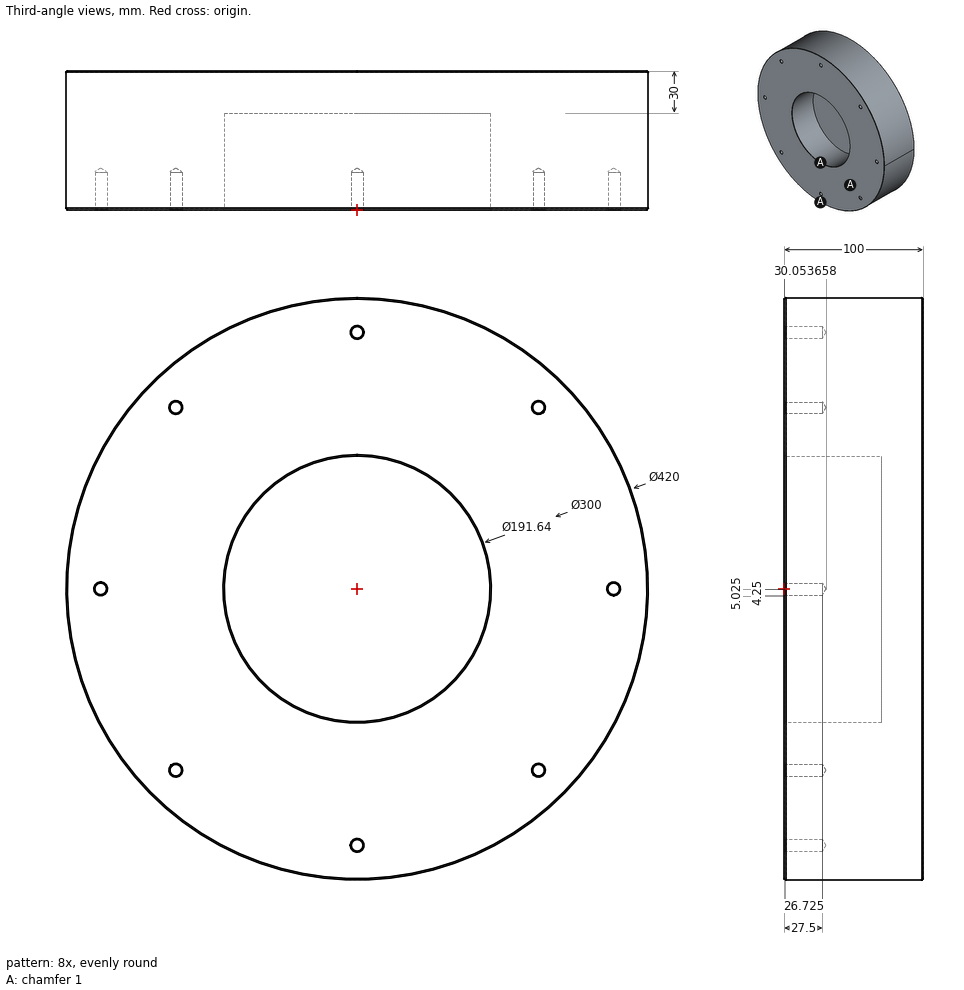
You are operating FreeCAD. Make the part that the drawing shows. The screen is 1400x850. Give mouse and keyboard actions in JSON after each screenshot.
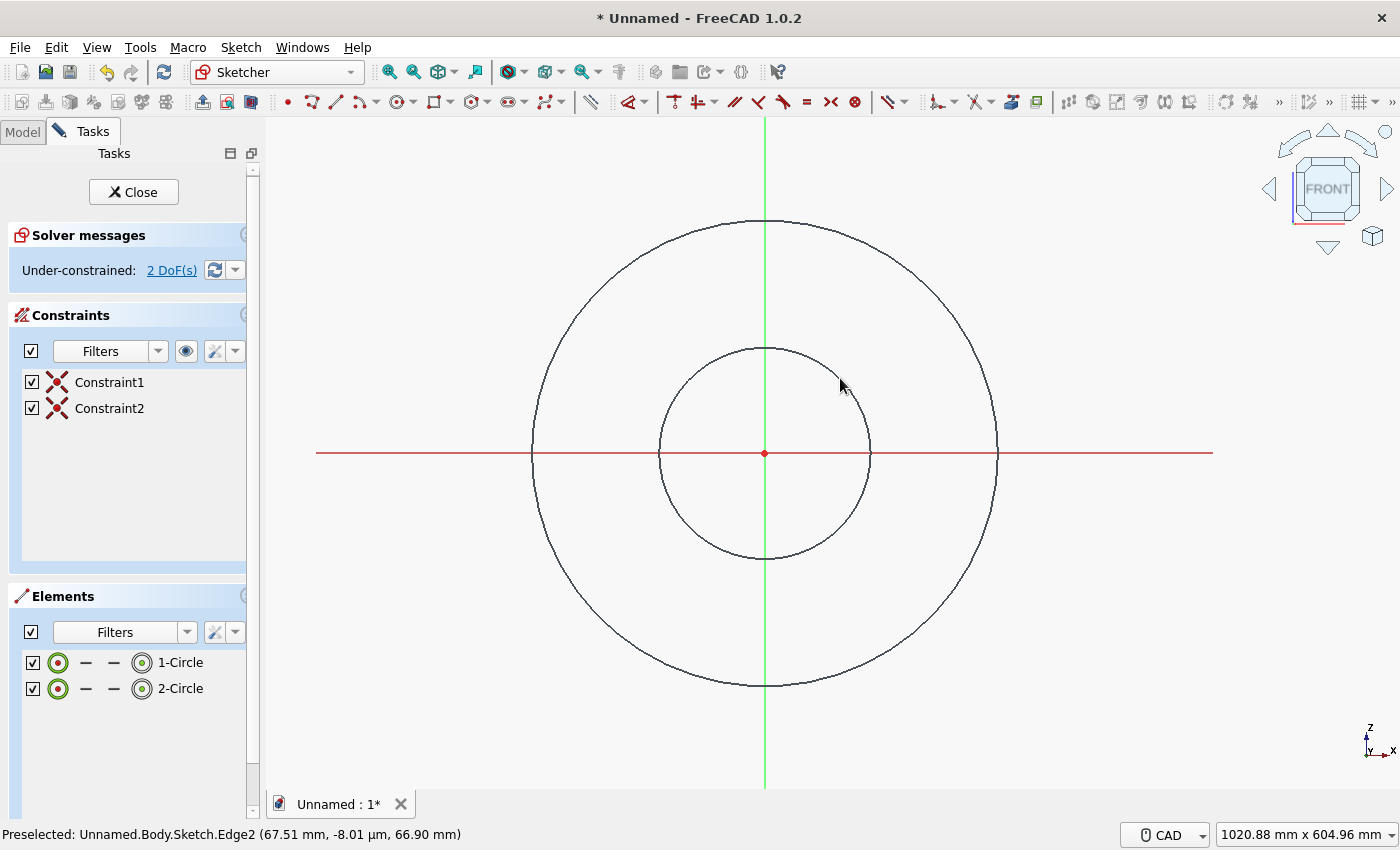
{"action": "left_click", "coordinate": [929, 288]}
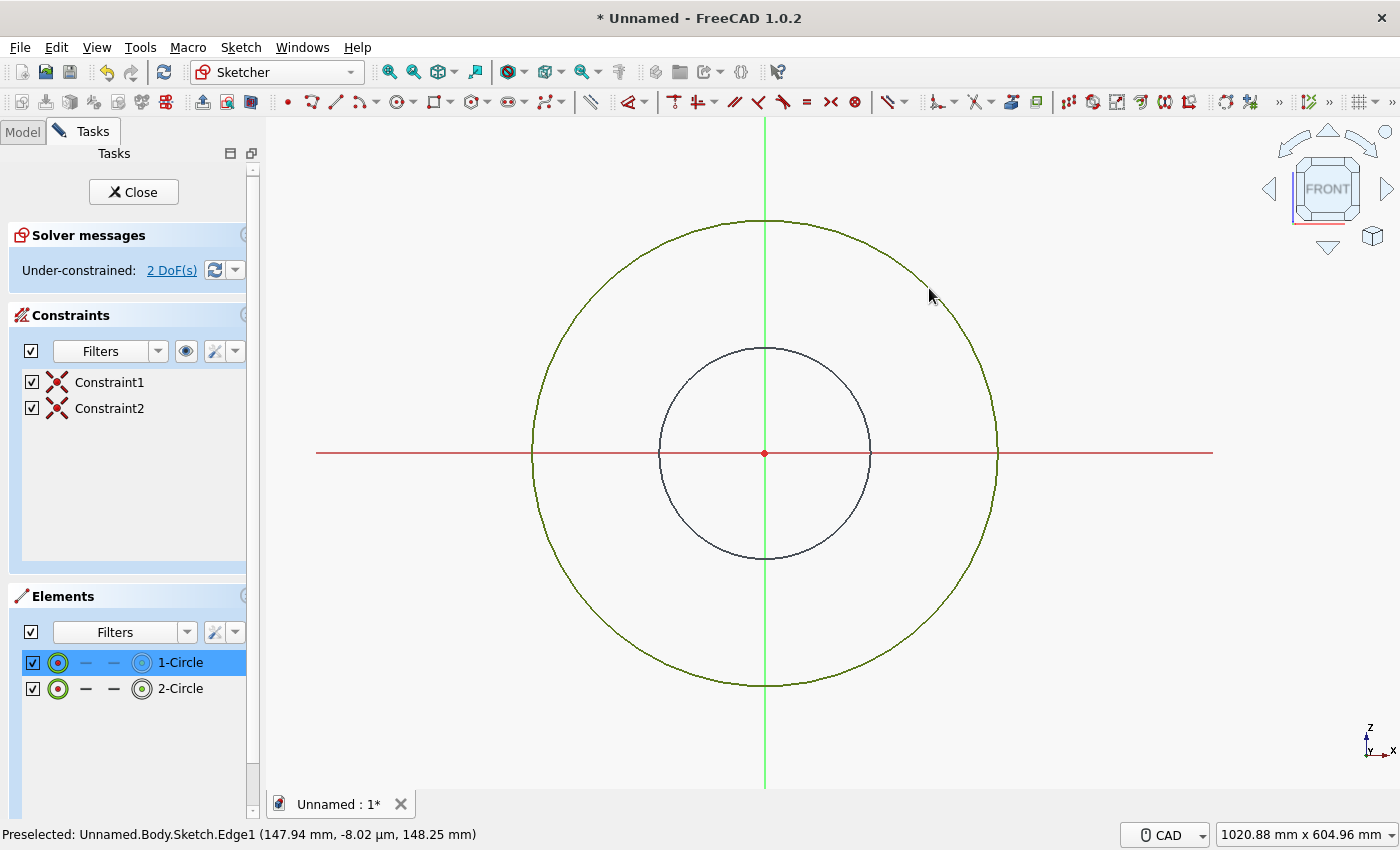
{"action": "key", "text": "k o"}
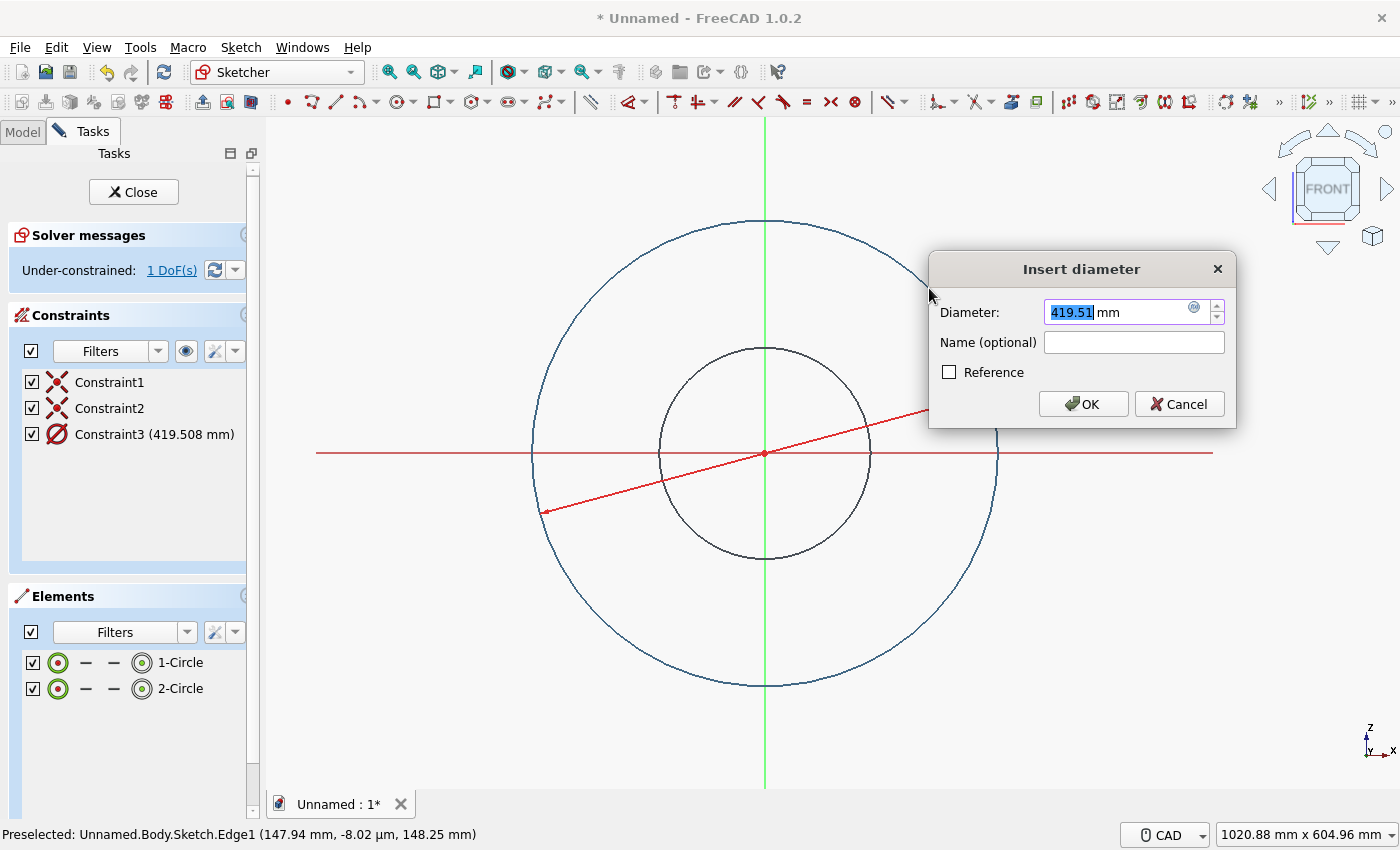
{"action": "type", "text": "420"}
{"action": "key", "text": "Return"}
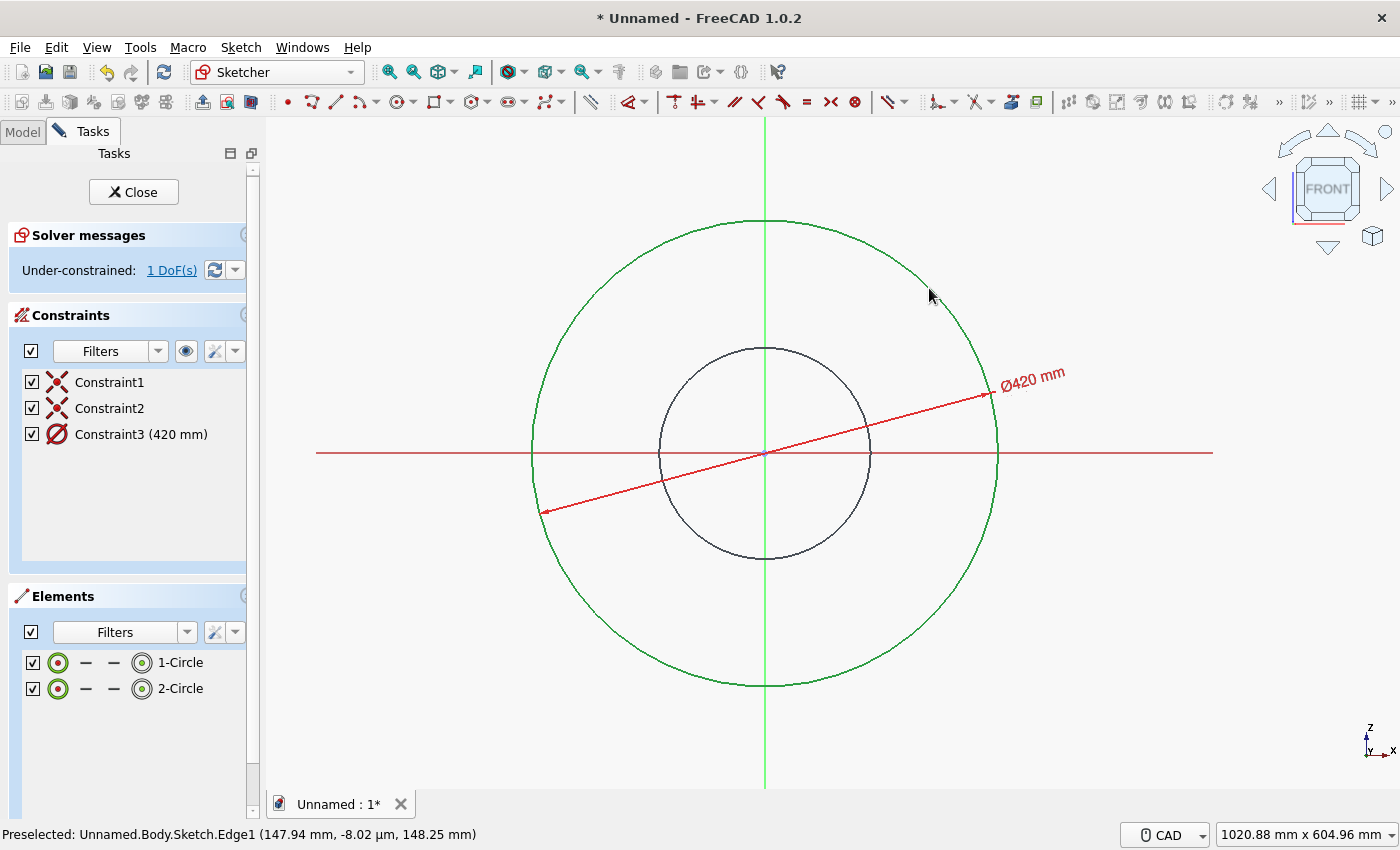
{"action": "left_click", "coordinate": [839, 378]}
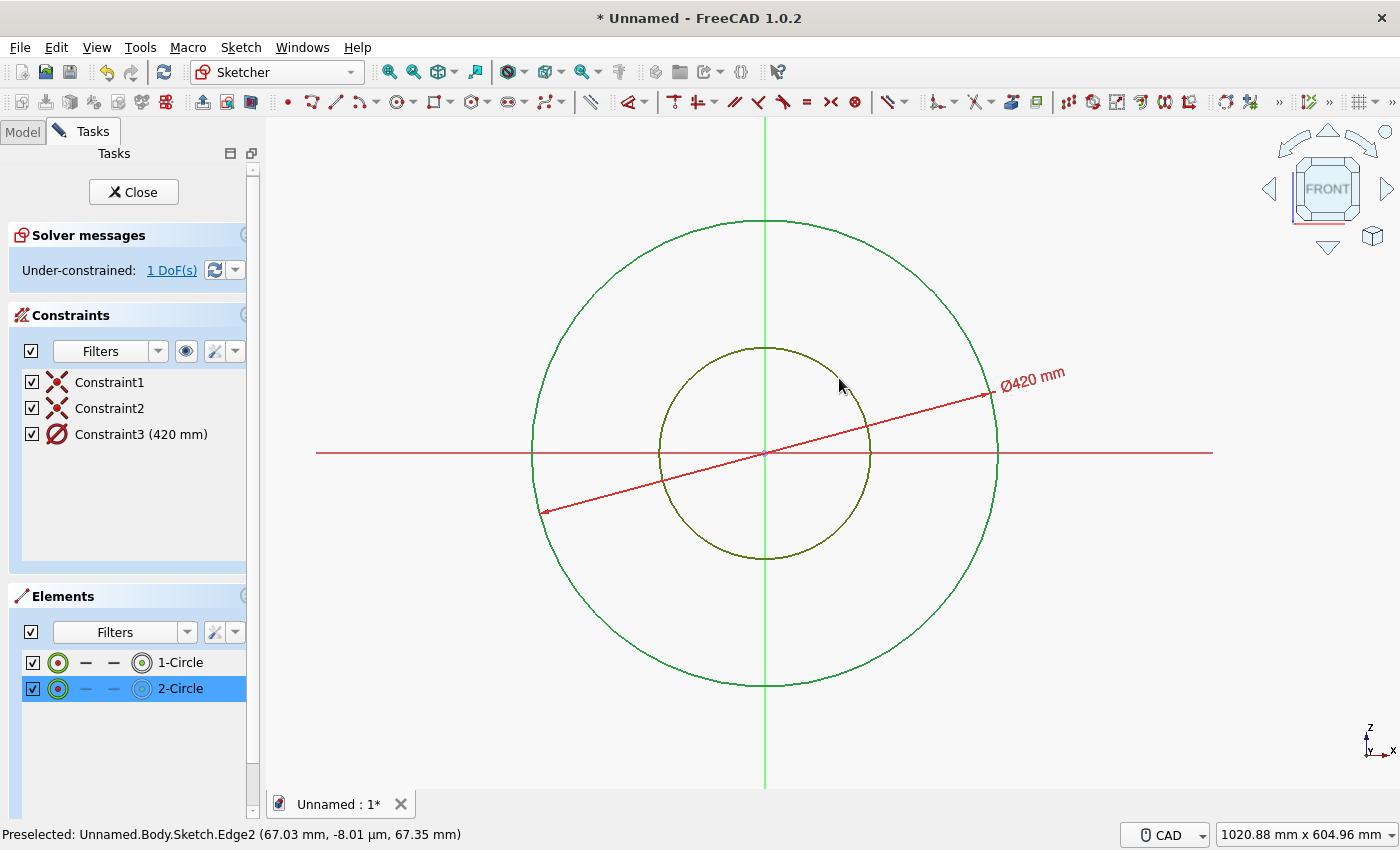
{"action": "key", "text": "k o"}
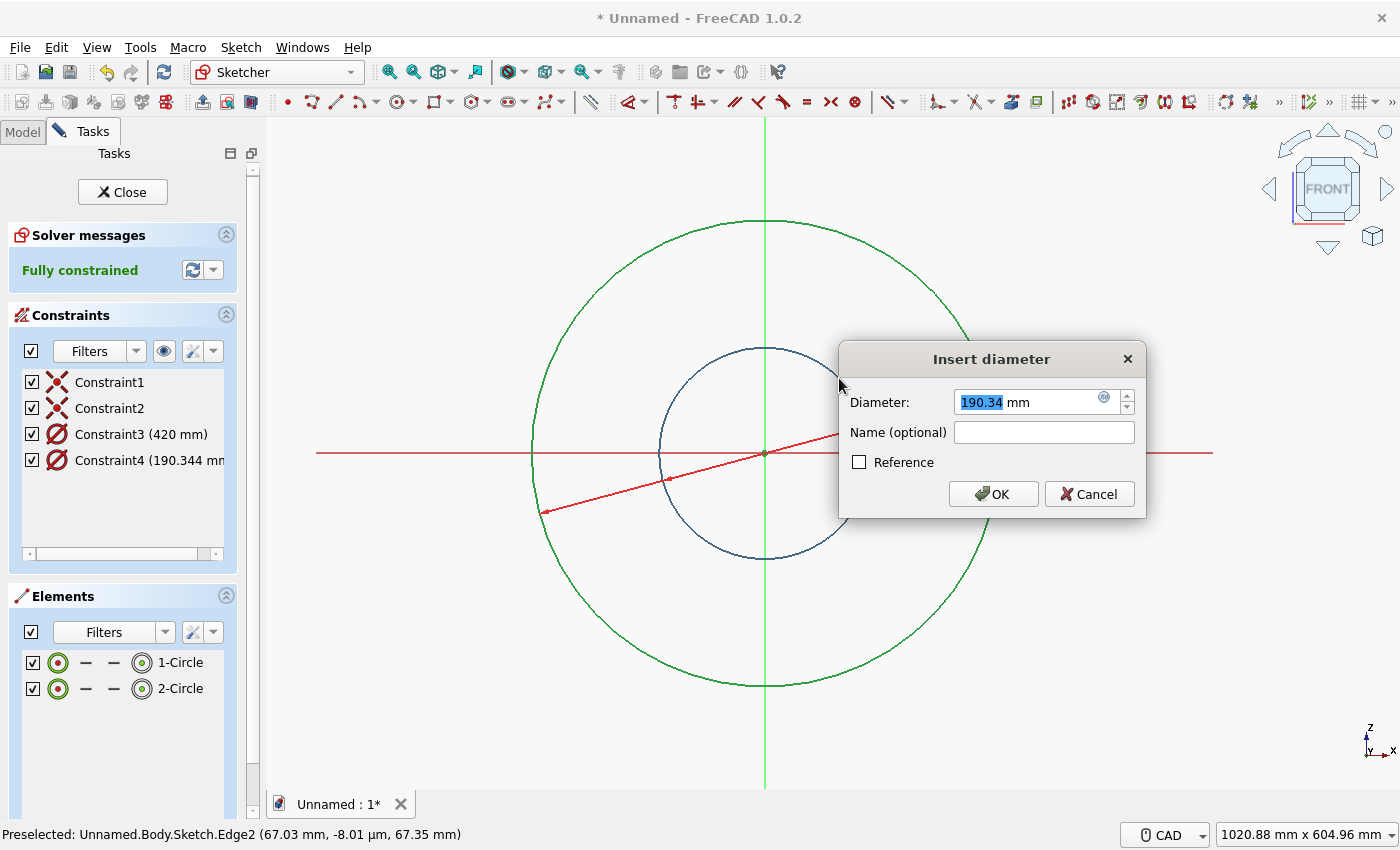
{"action": "type", "text": "191.64"}
{"action": "key", "text": "Return"}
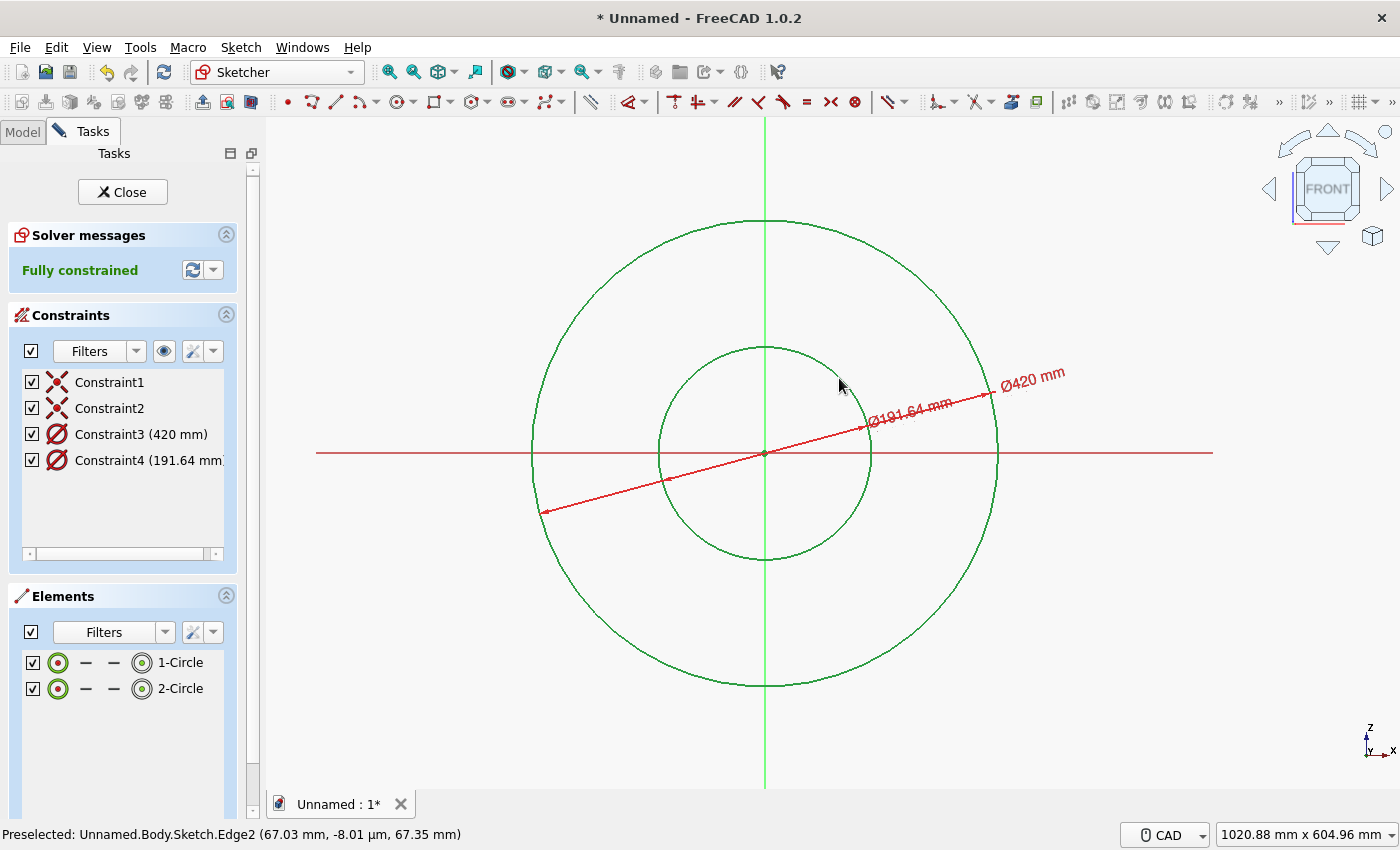
{"action": "left_click", "coordinate": [123, 192]}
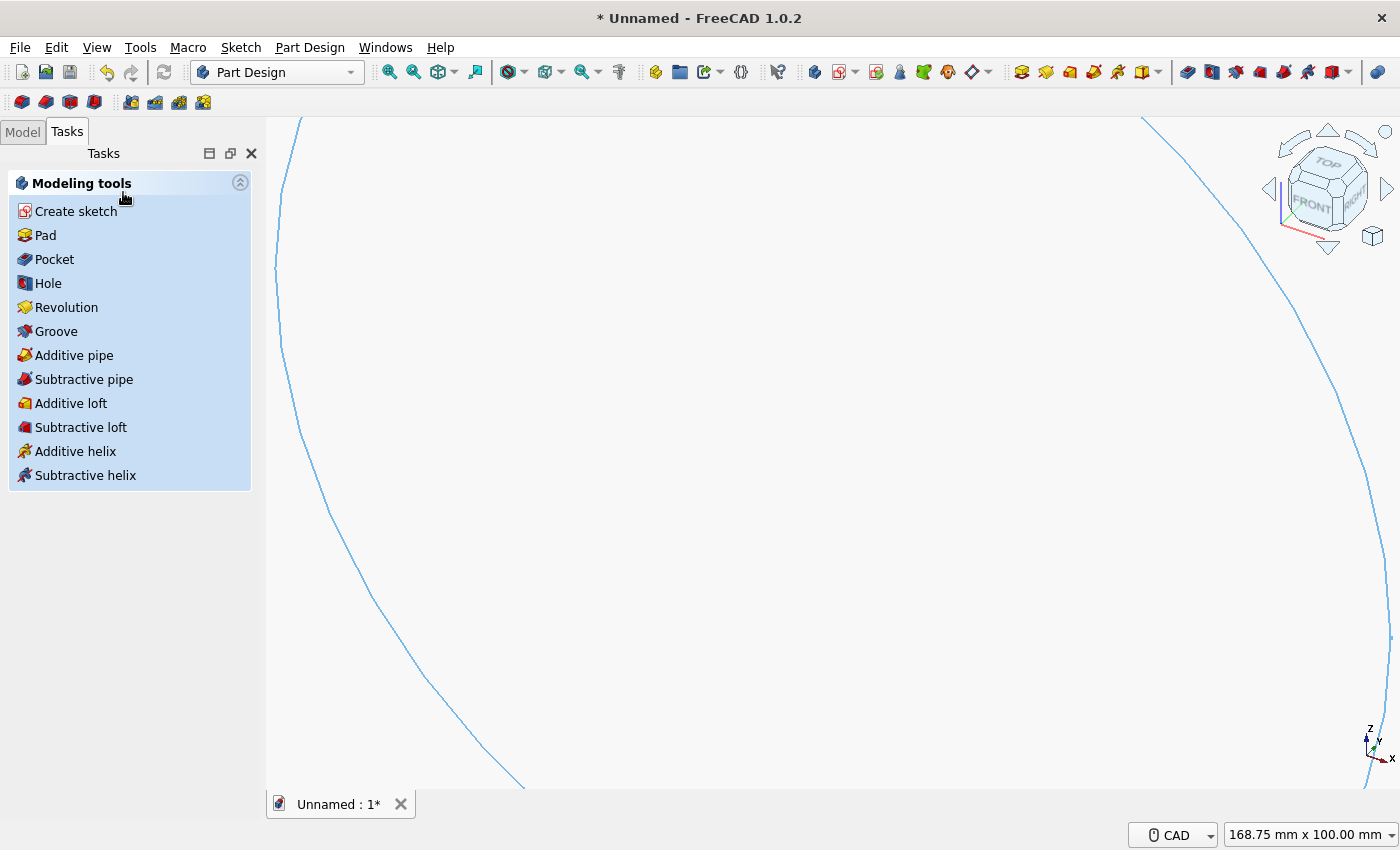
{"action": "left_click", "coordinate": [1022, 72]}